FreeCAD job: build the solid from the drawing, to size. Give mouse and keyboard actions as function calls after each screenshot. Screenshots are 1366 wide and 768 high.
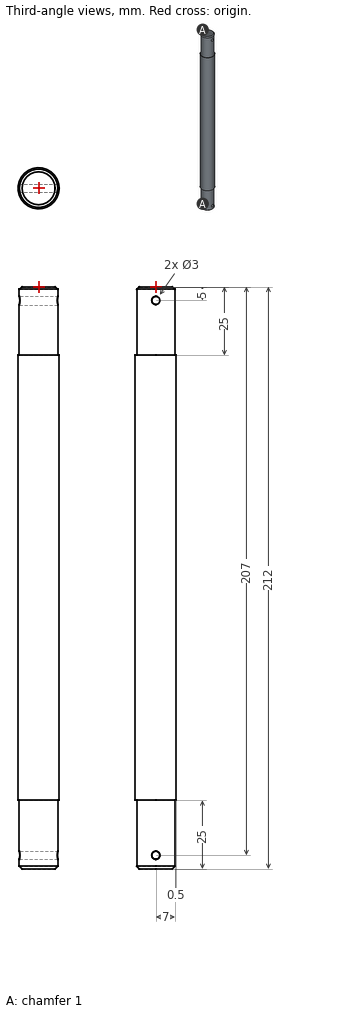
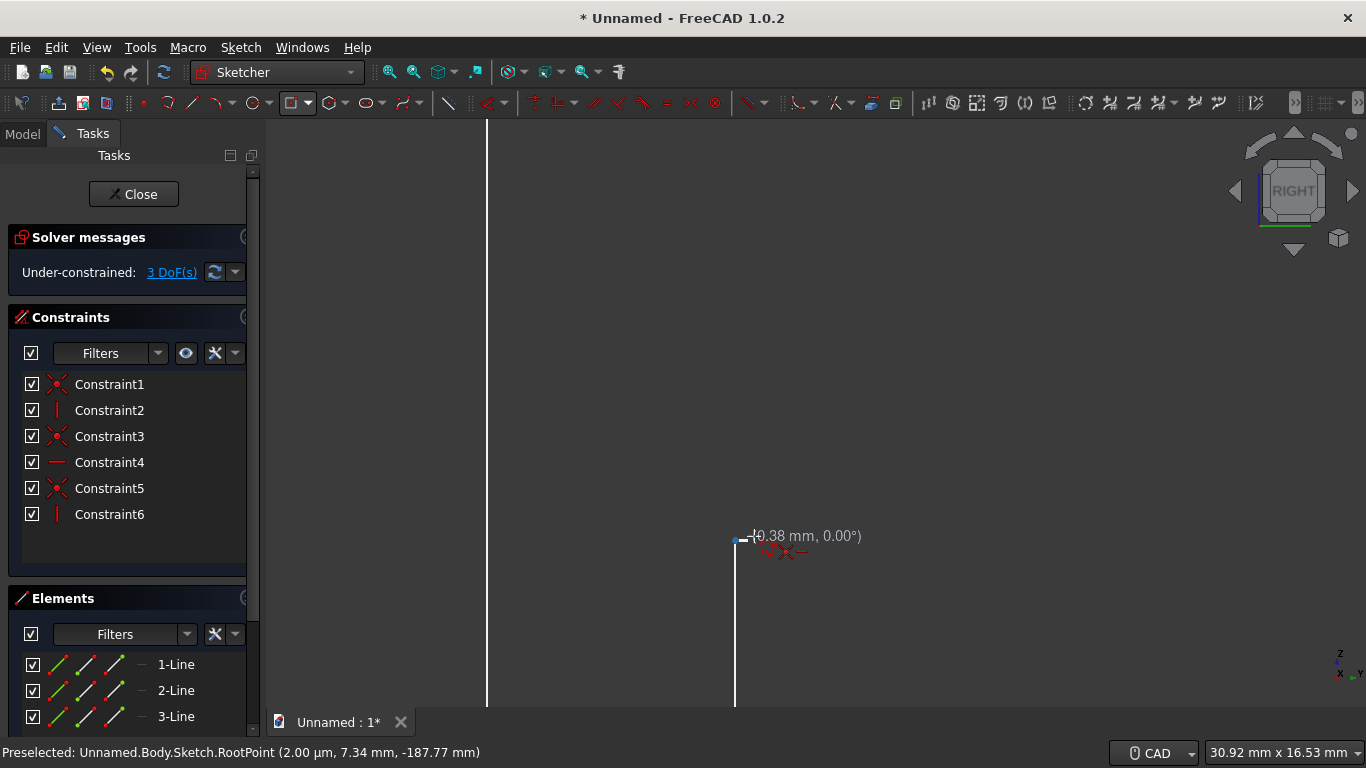
click(754, 527)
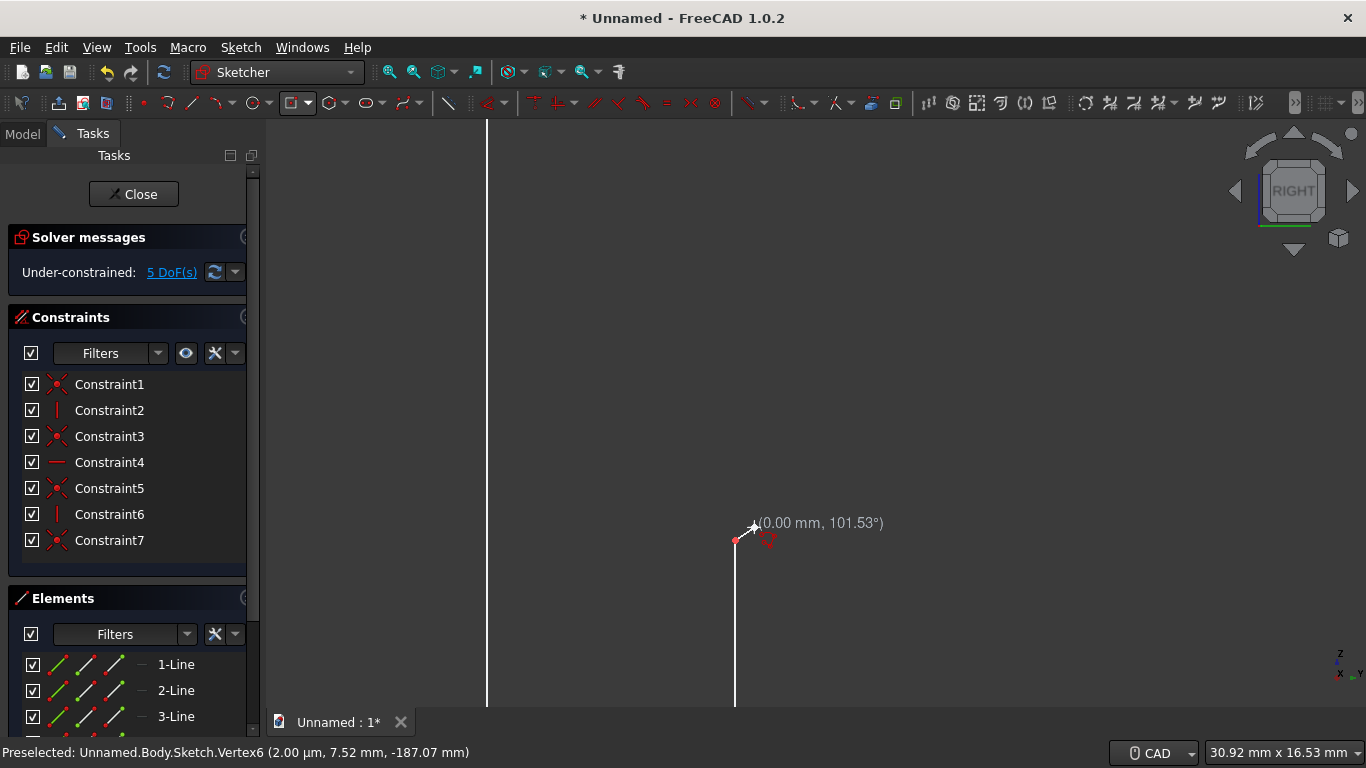
scroll(754, 558, down, 15)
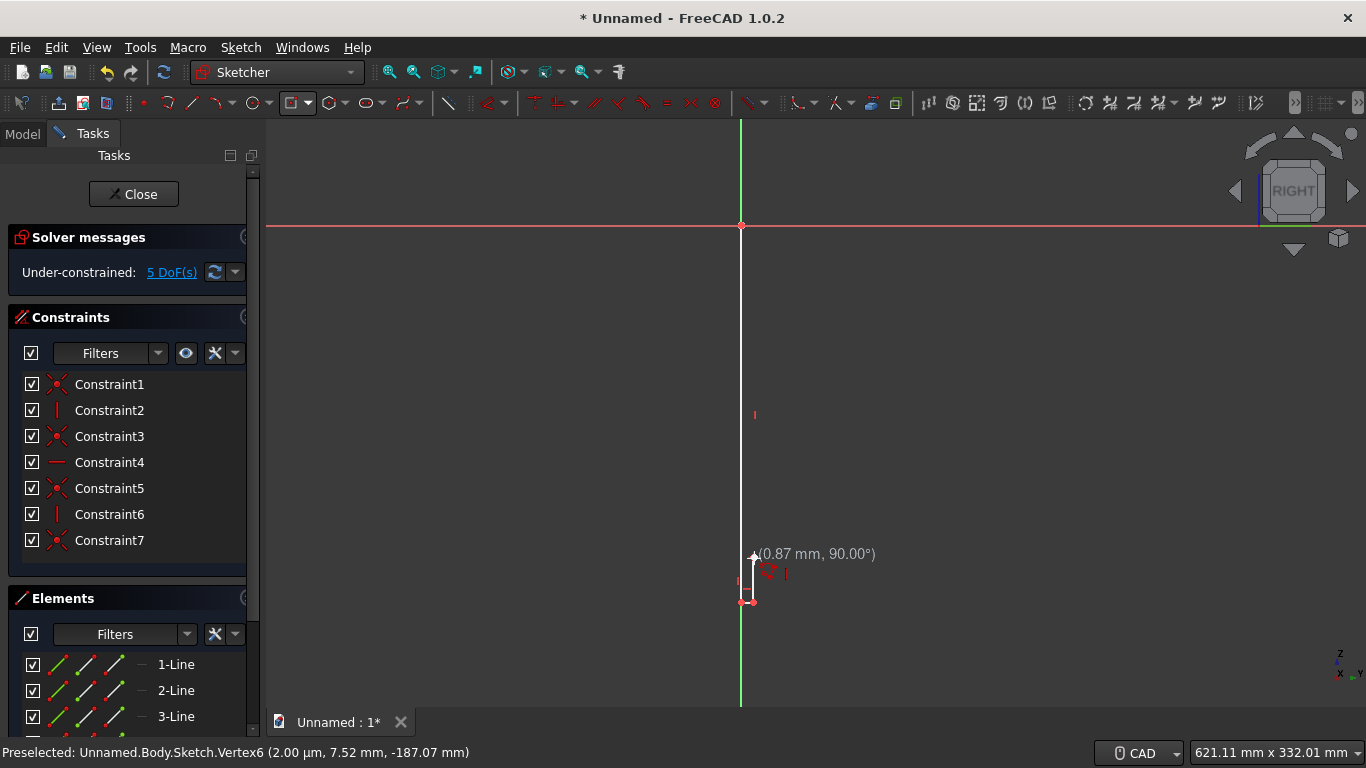
click(754, 270)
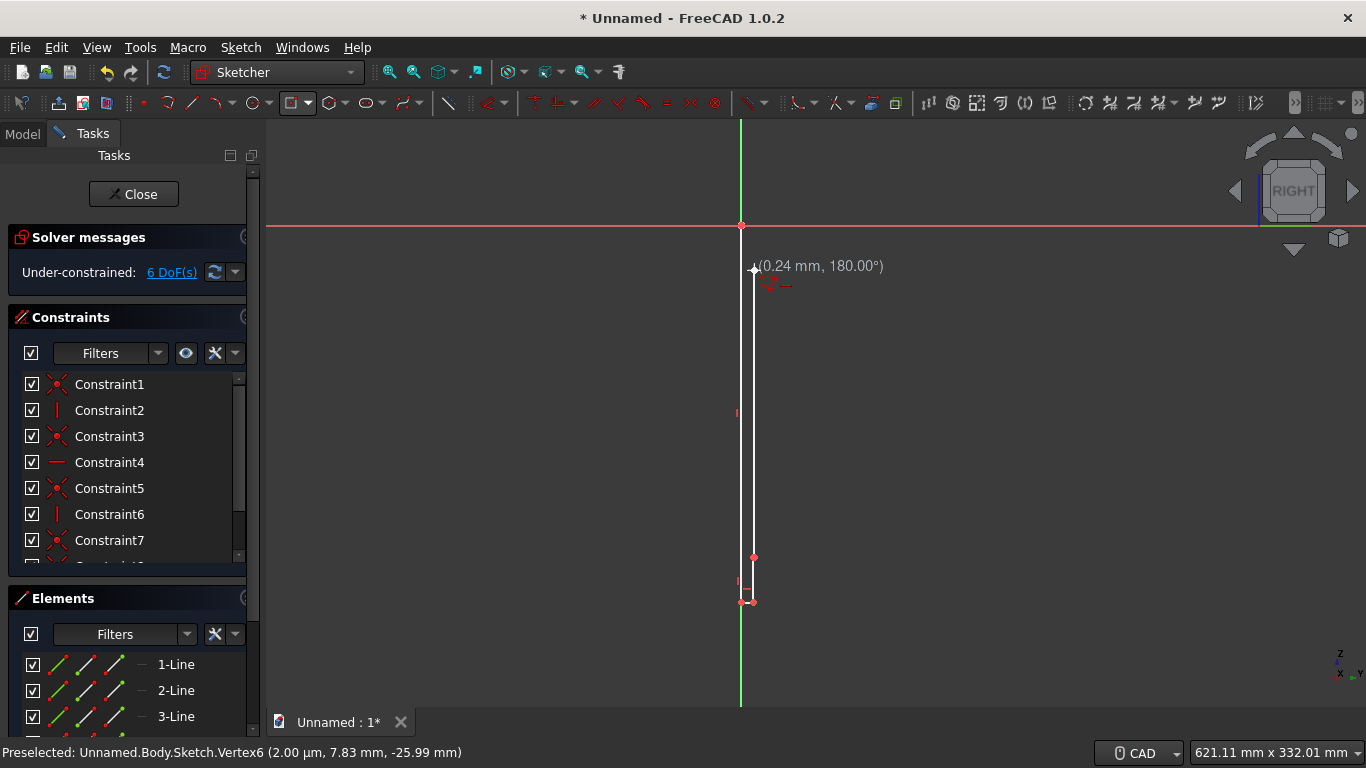
scroll(754, 270, up, 15)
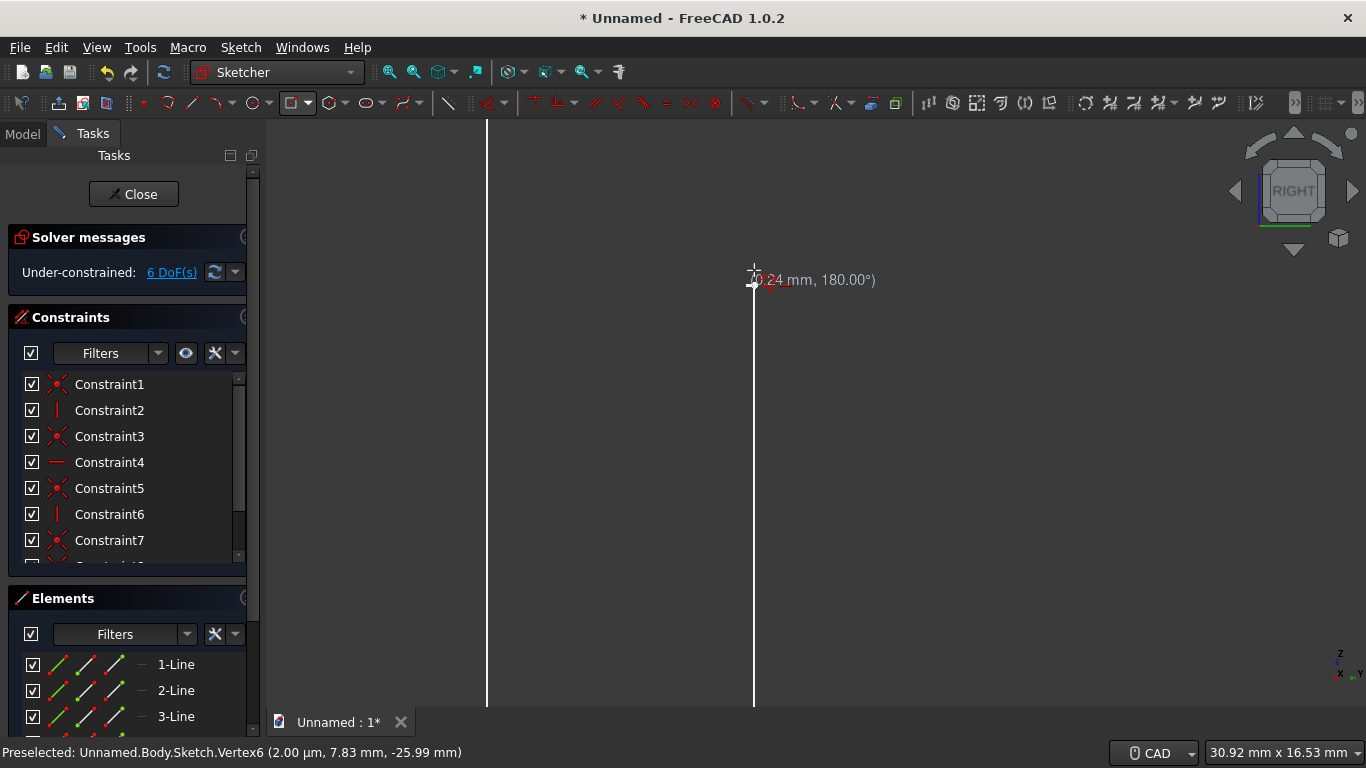
click(736, 265)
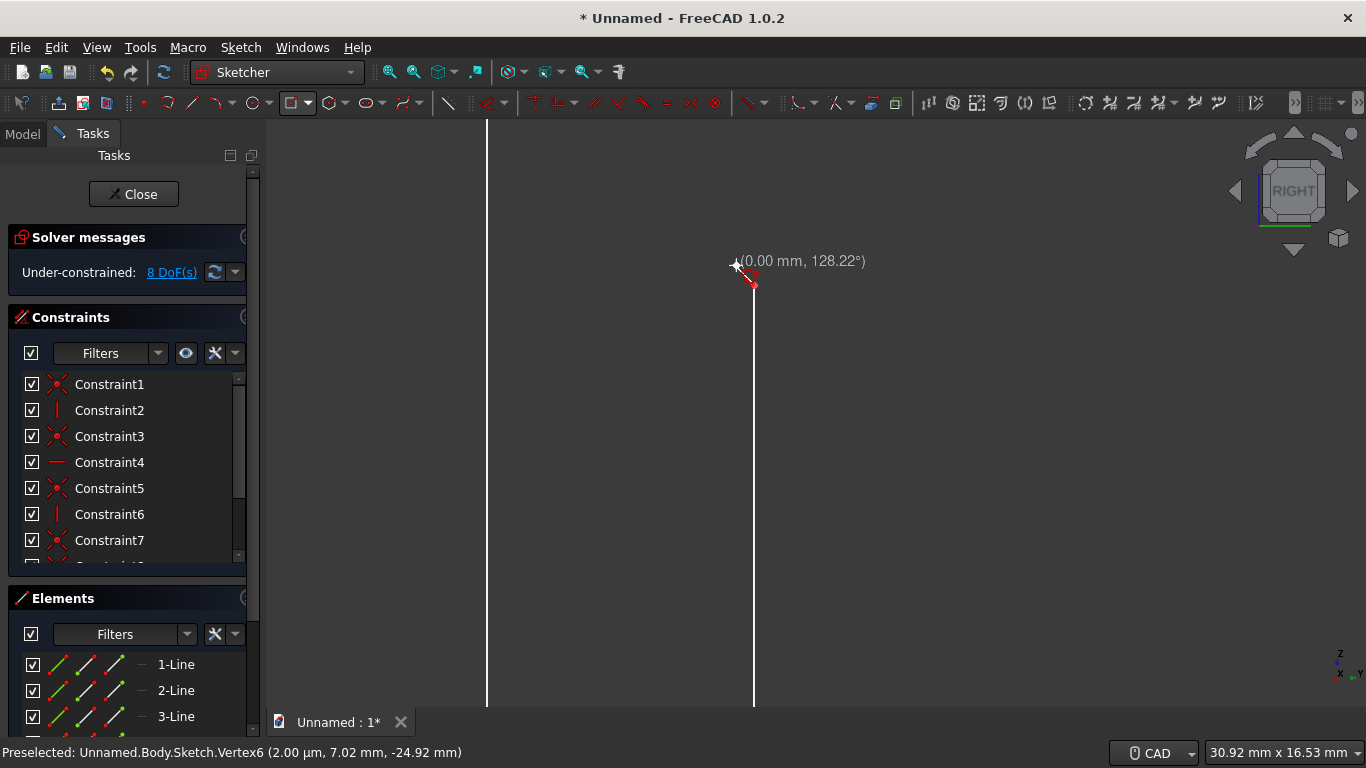
scroll(754, 270, down, 15)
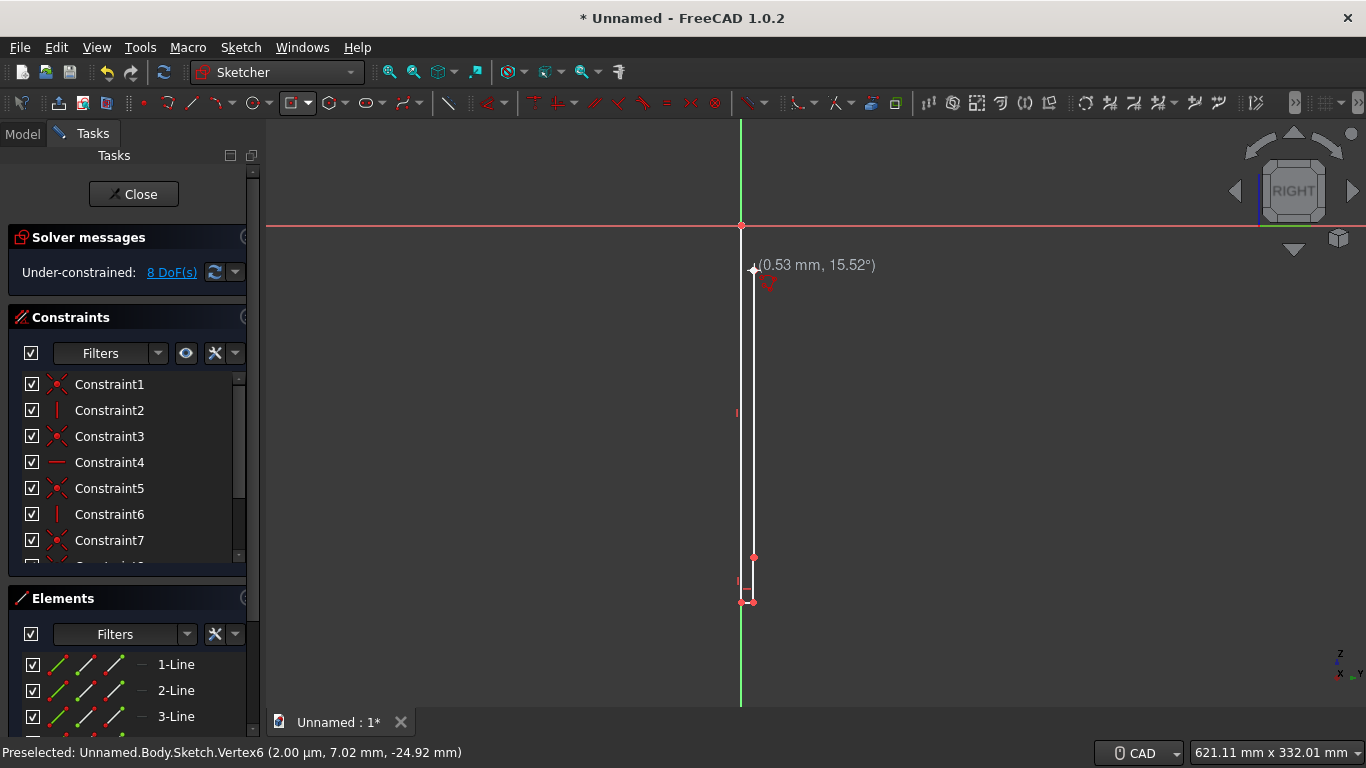
scroll(754, 226, up, 2)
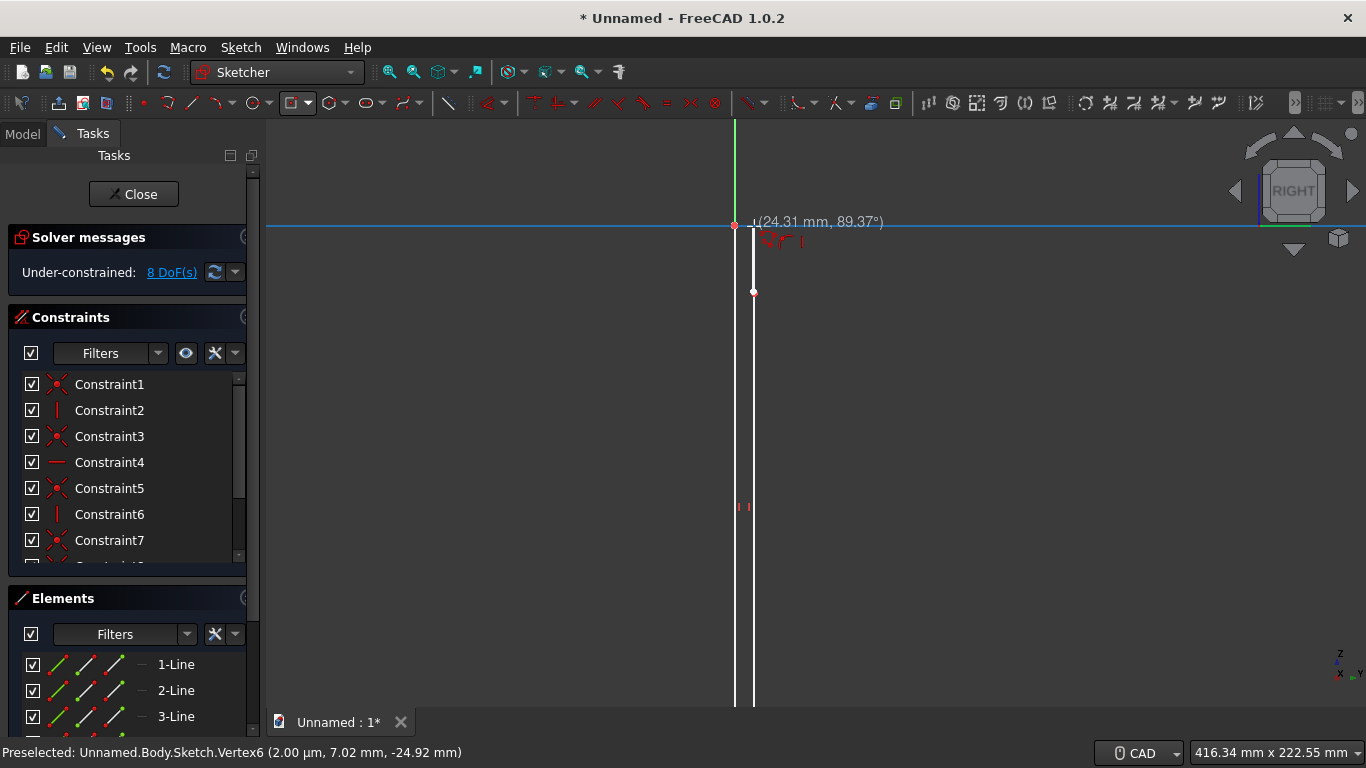
click(753, 235)
click(735, 226)
key(Escape)
key(Escape)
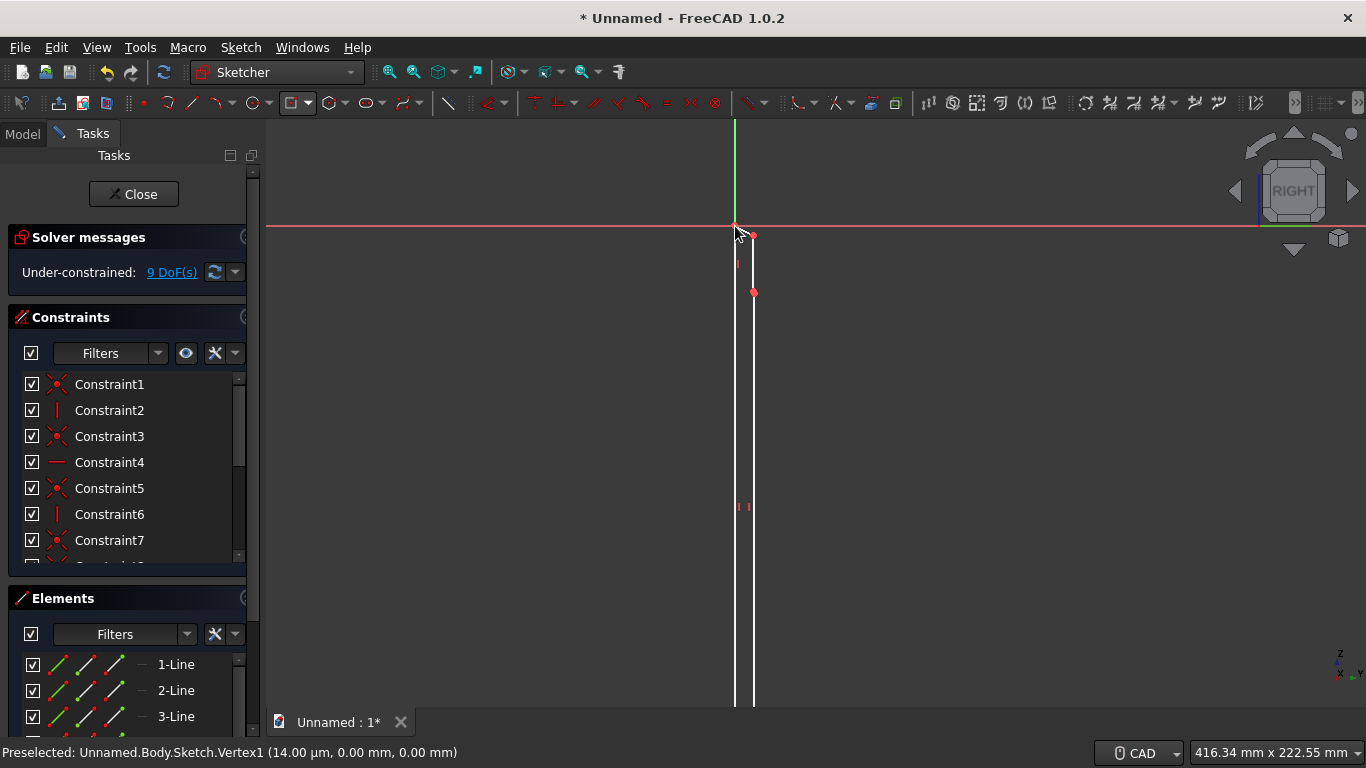
scroll(754, 224, down, 2)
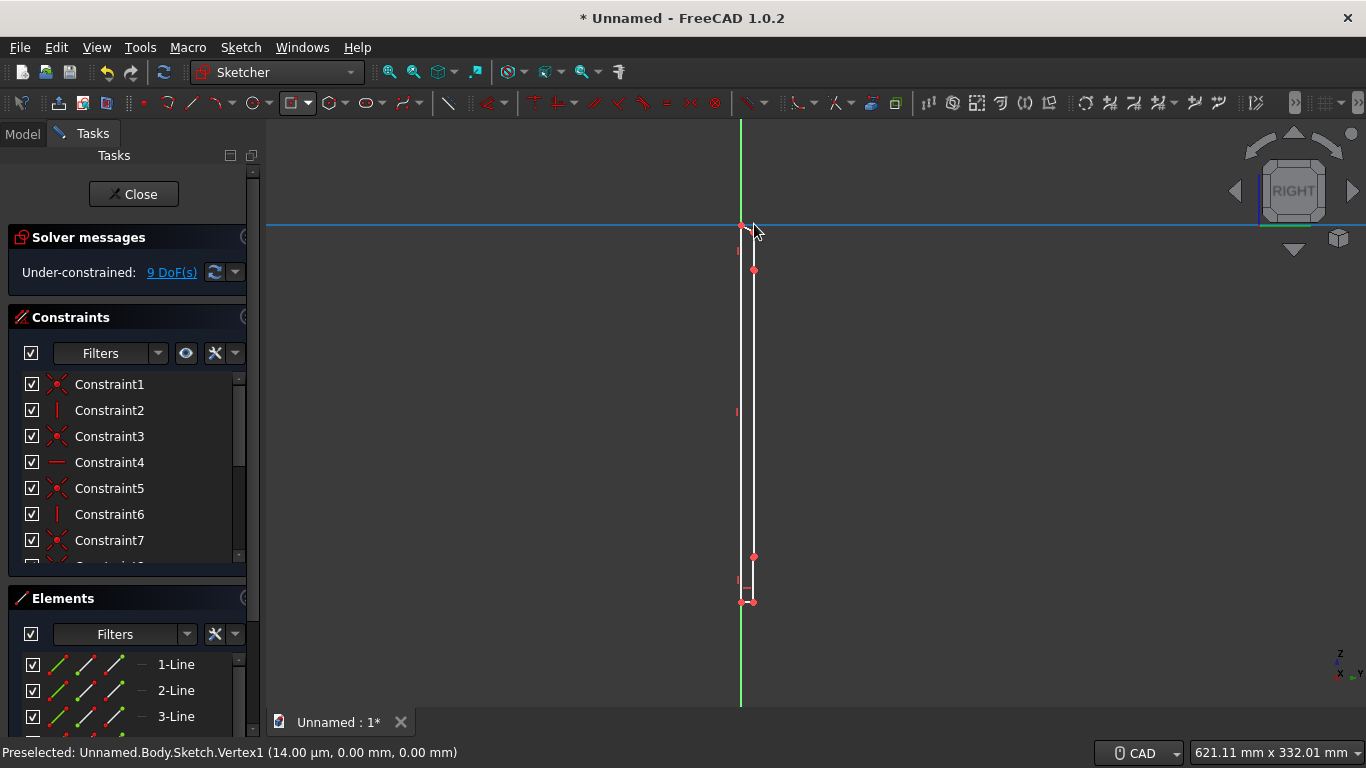
scroll(754, 557, up, 14)